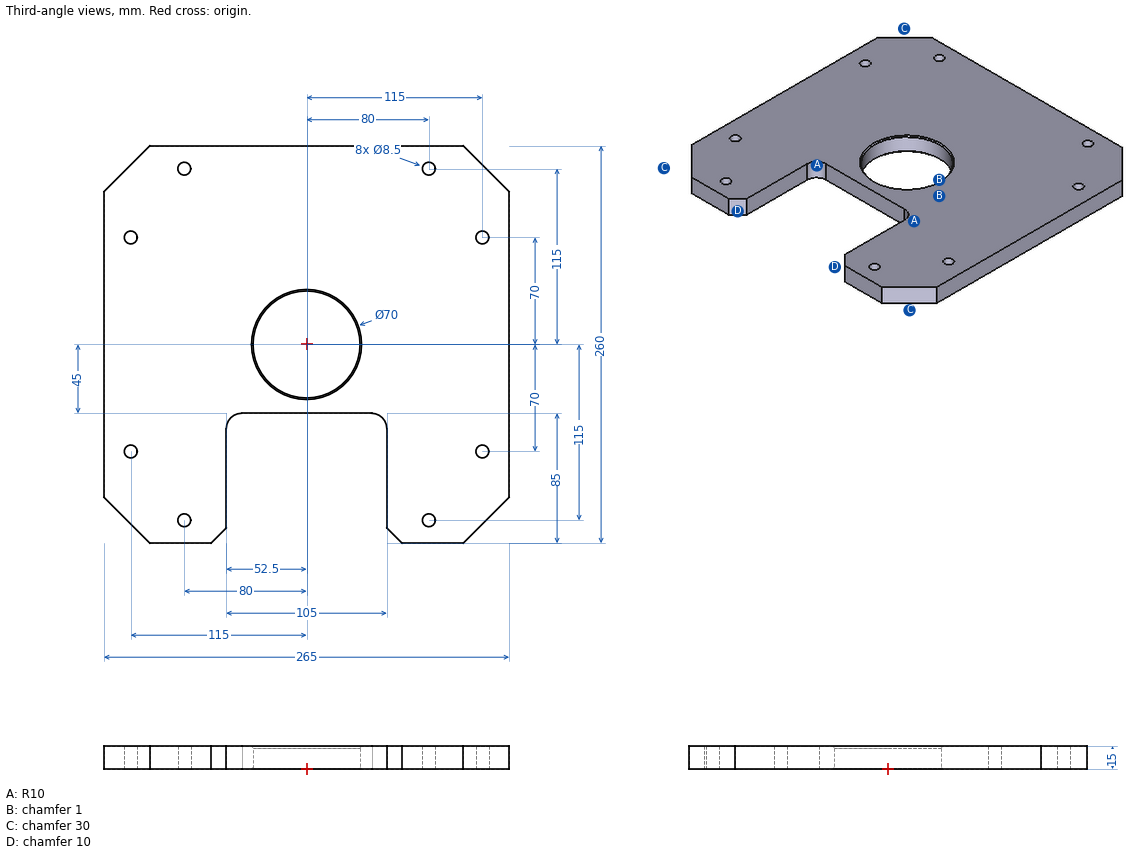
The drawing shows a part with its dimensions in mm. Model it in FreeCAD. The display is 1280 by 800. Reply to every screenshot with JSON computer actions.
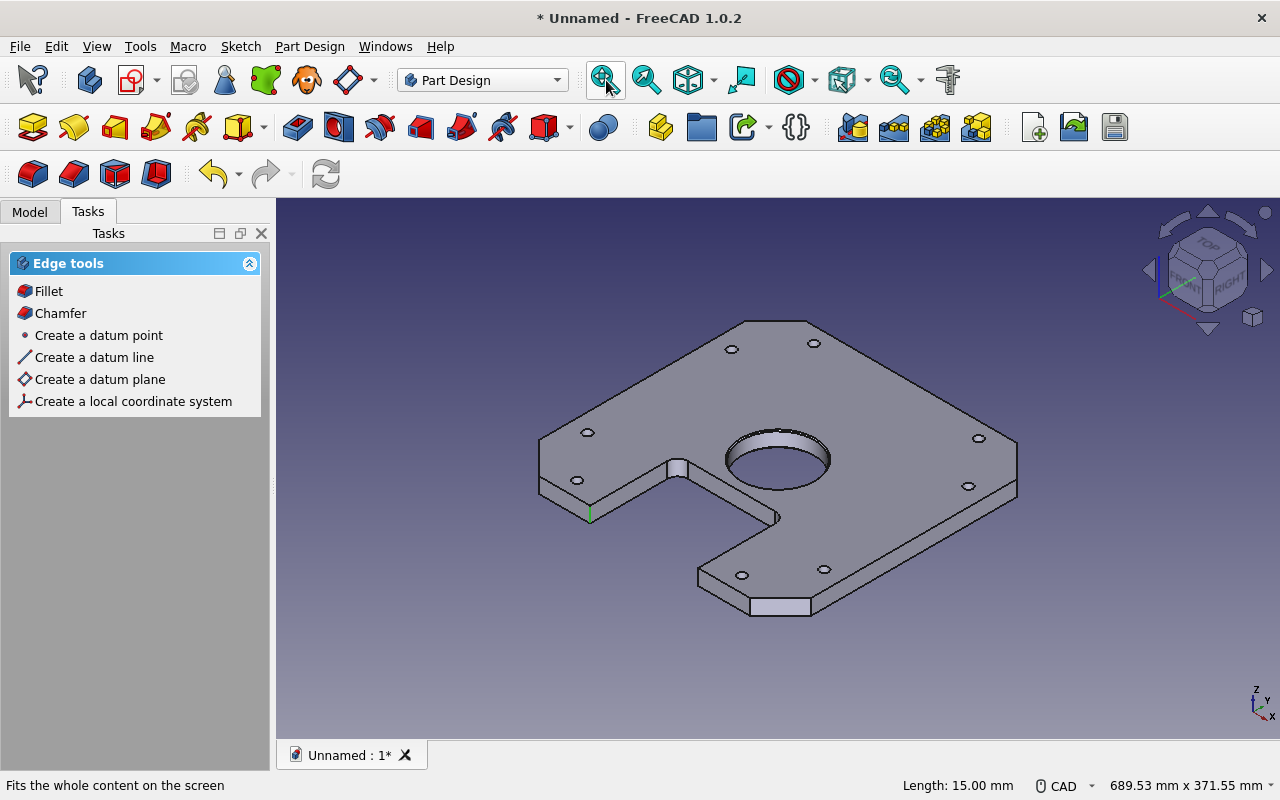
{"action": "key", "text": "2"}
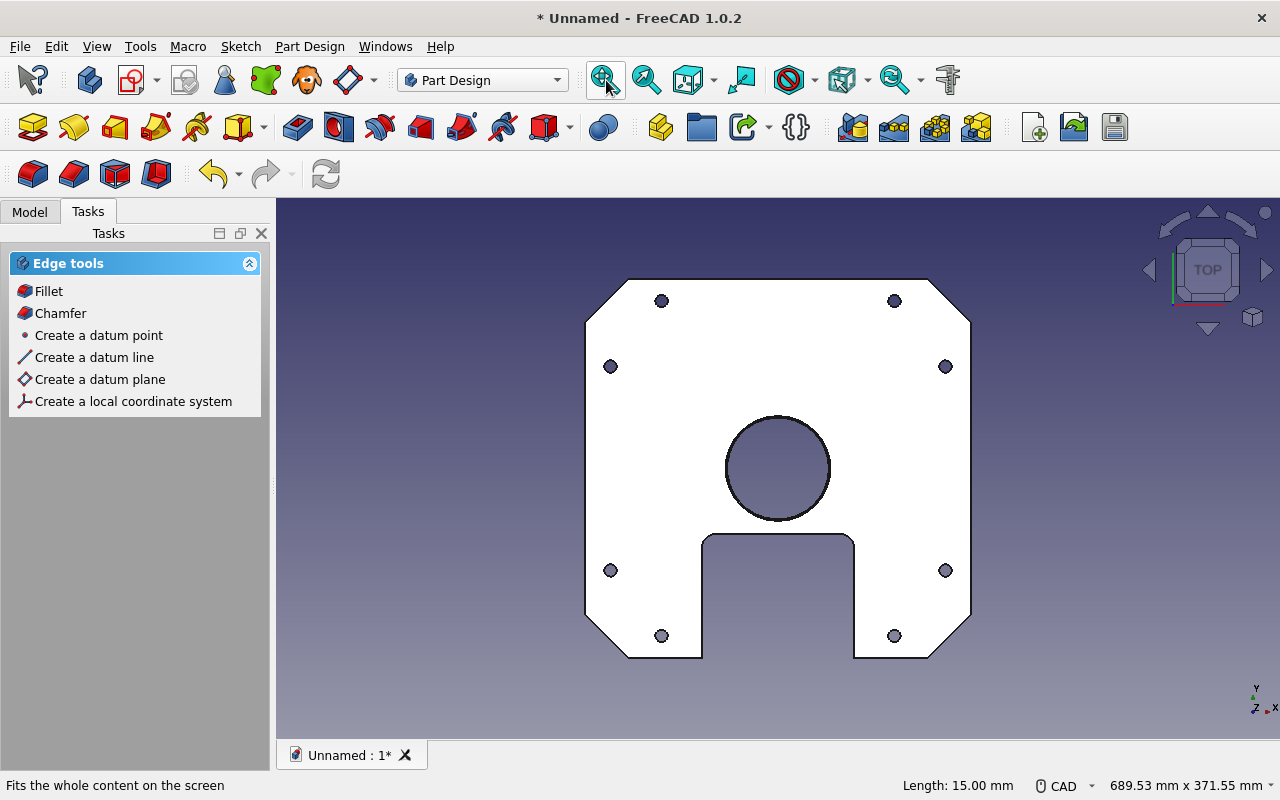
{"action": "scroll", "coordinate": [854, 657], "scroll_direction": "up", "scroll_amount": 4}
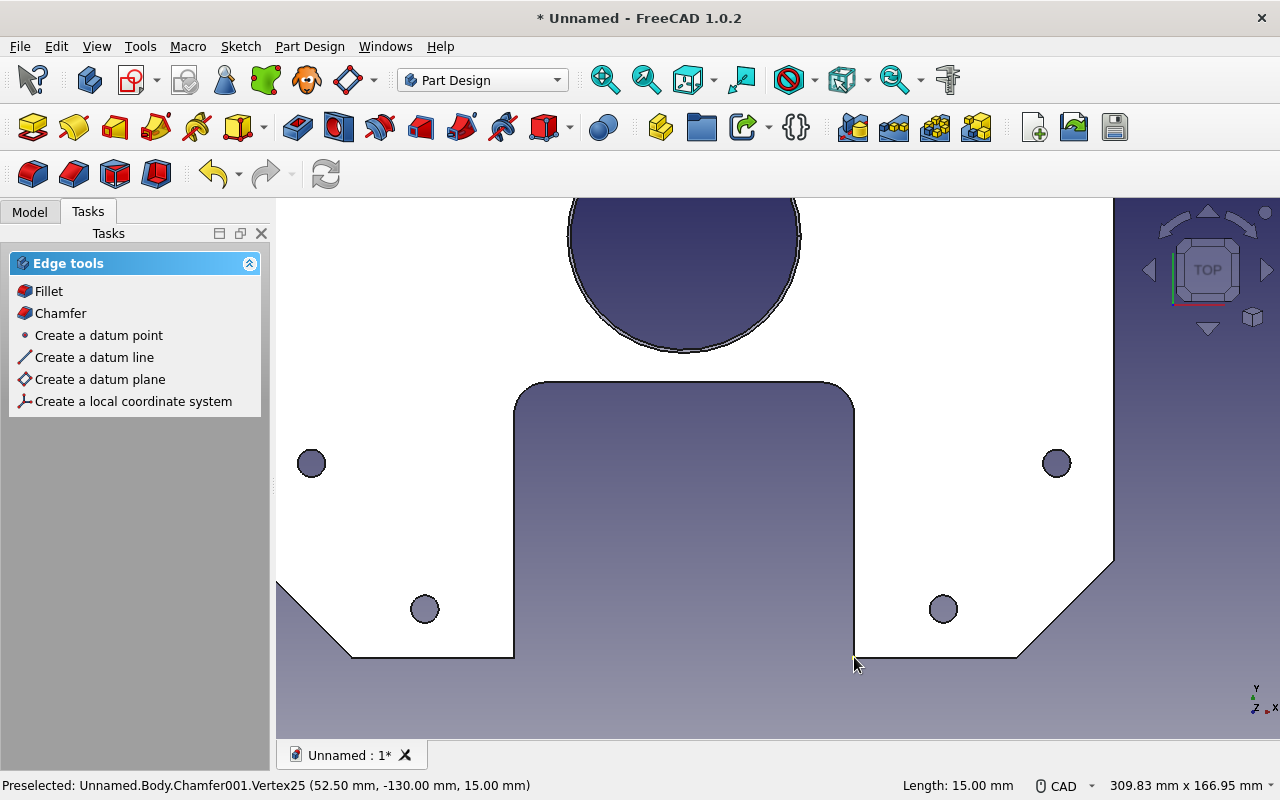
{"action": "left_click", "coordinate": [606, 80]}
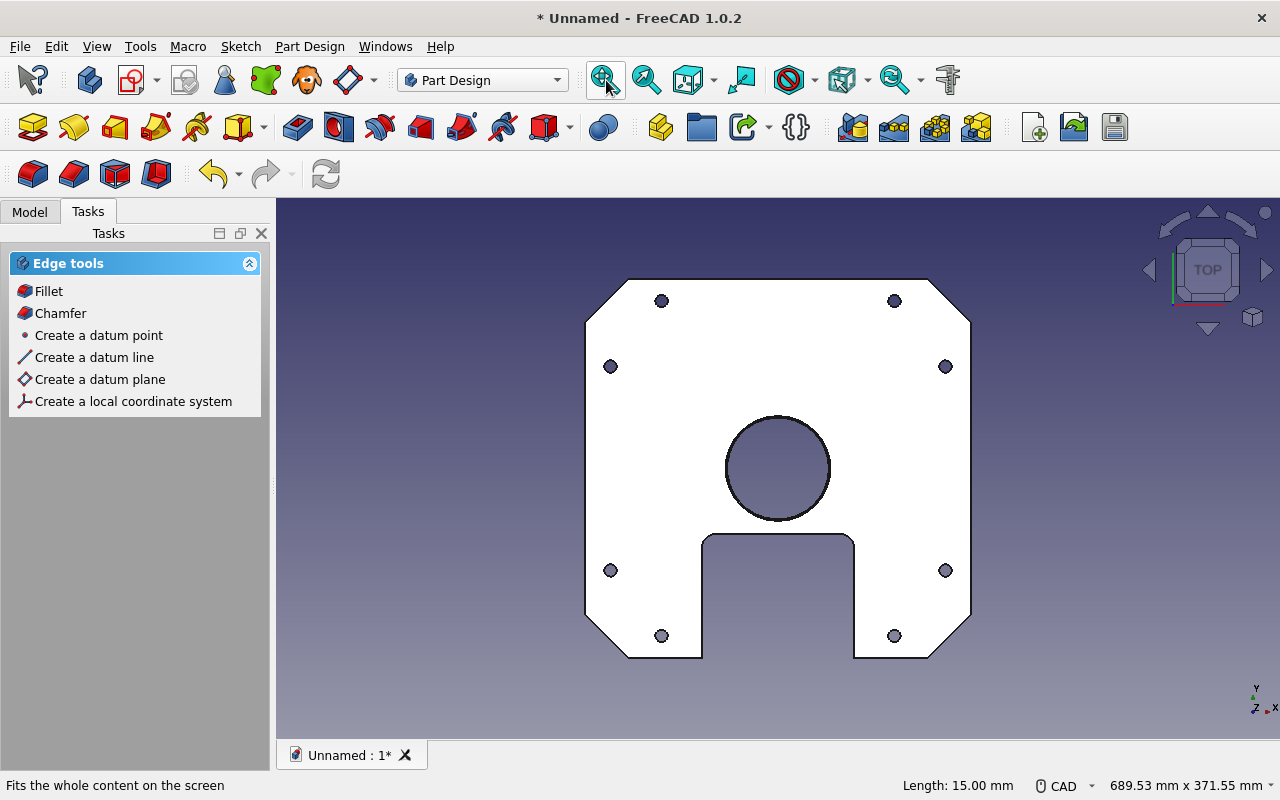
{"action": "key", "text": "1"}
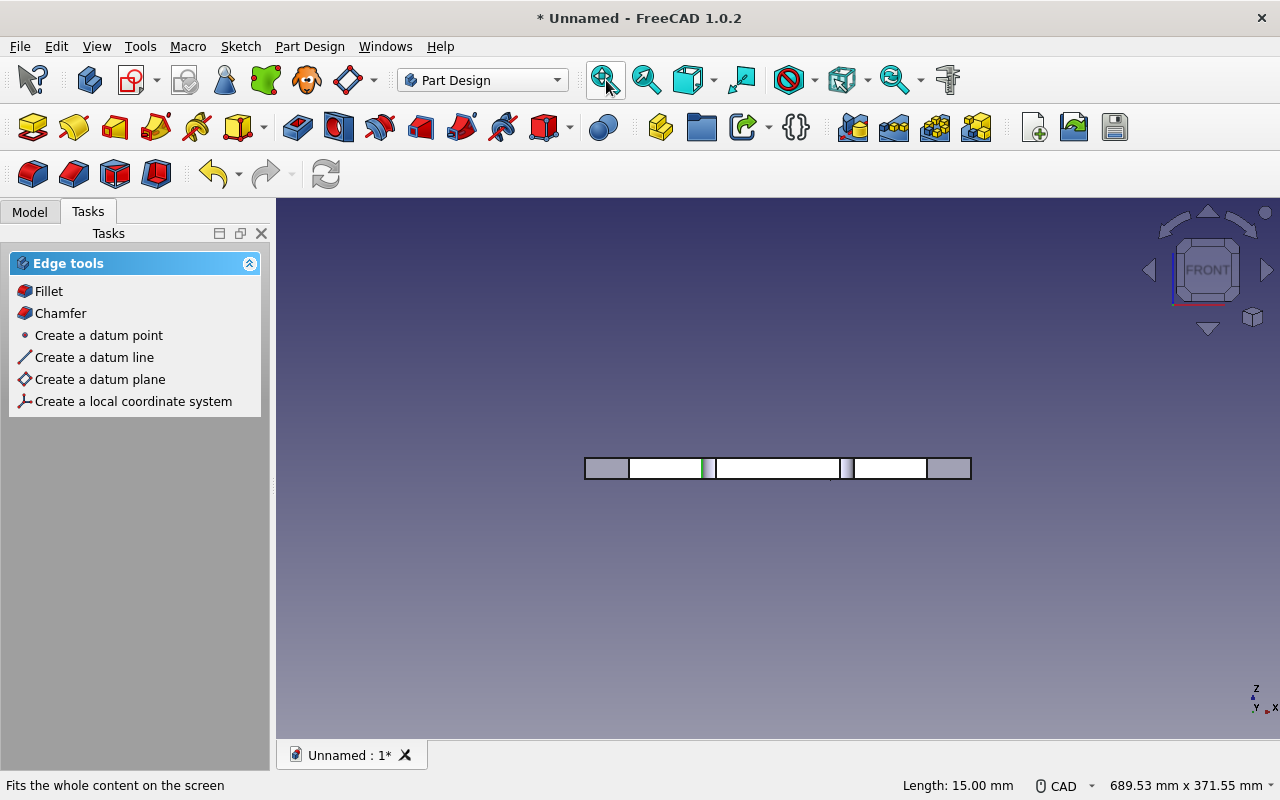
{"action": "key", "text": "v f"}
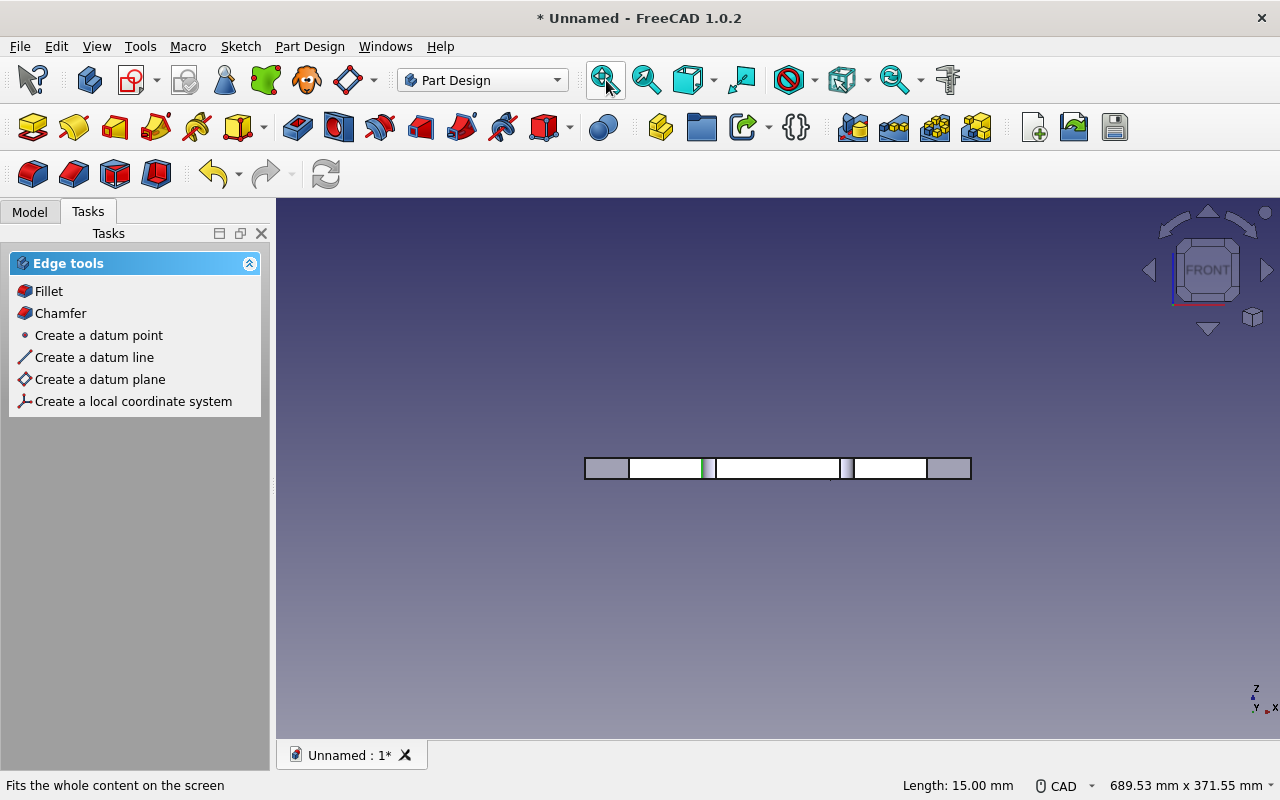
{"action": "left_click", "coordinate": [854, 468], "text": "ctrl"}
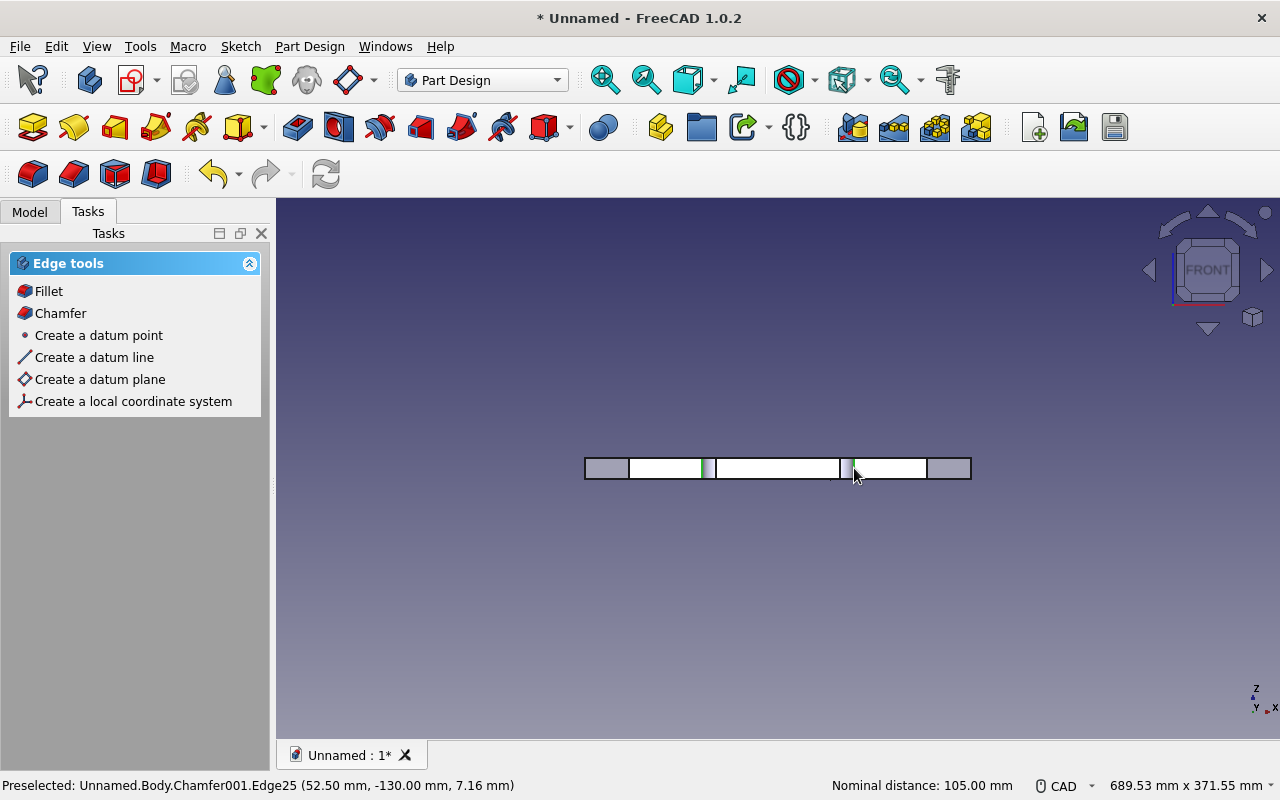
{"action": "left_click", "coordinate": [74, 174]}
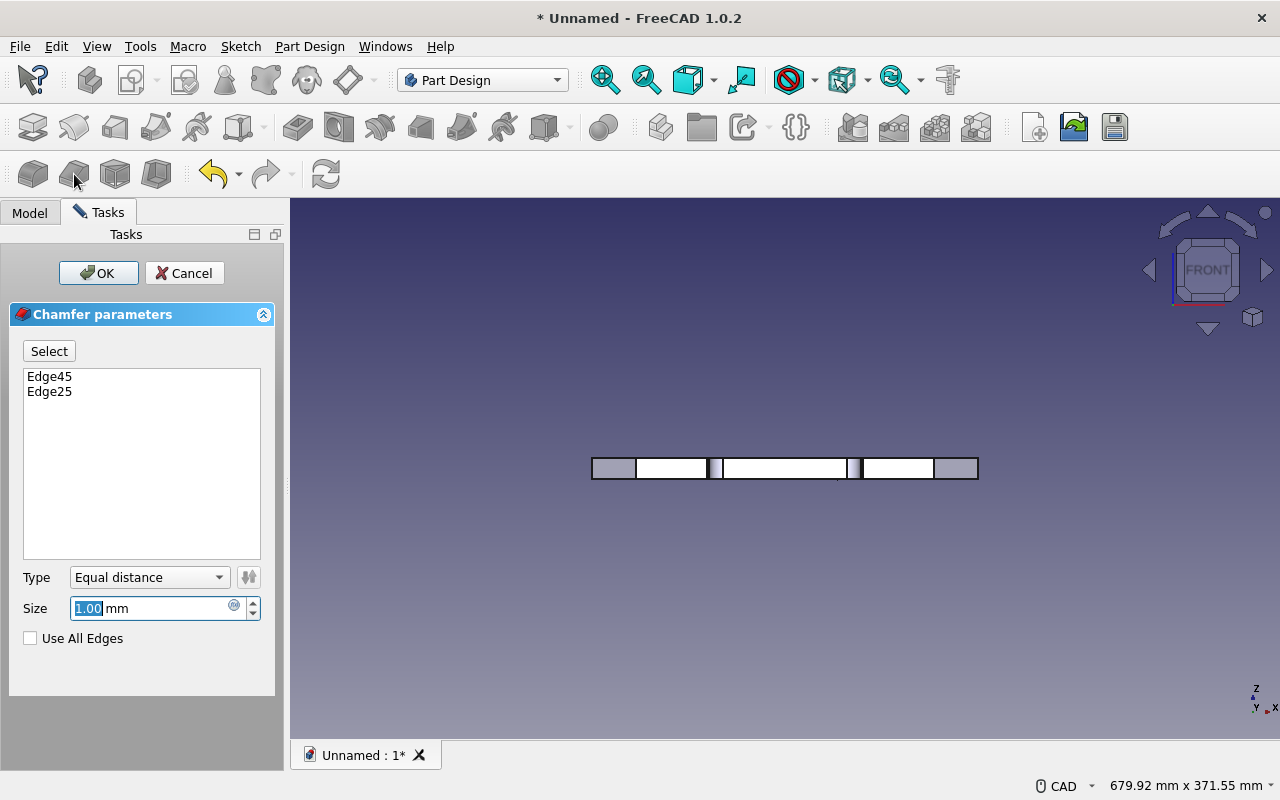
{"action": "type", "text": "10"}
{"action": "key", "text": "Tab"}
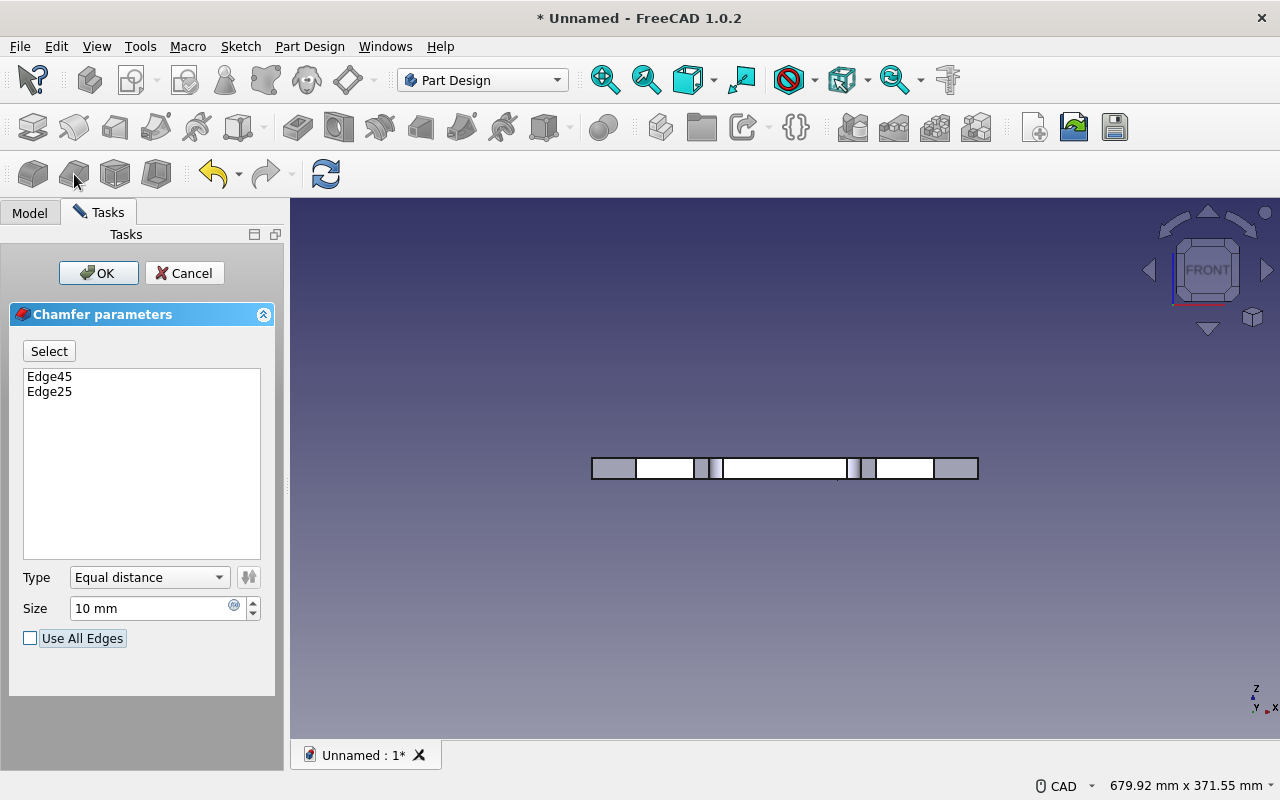
{"action": "left_click", "coordinate": [99, 273]}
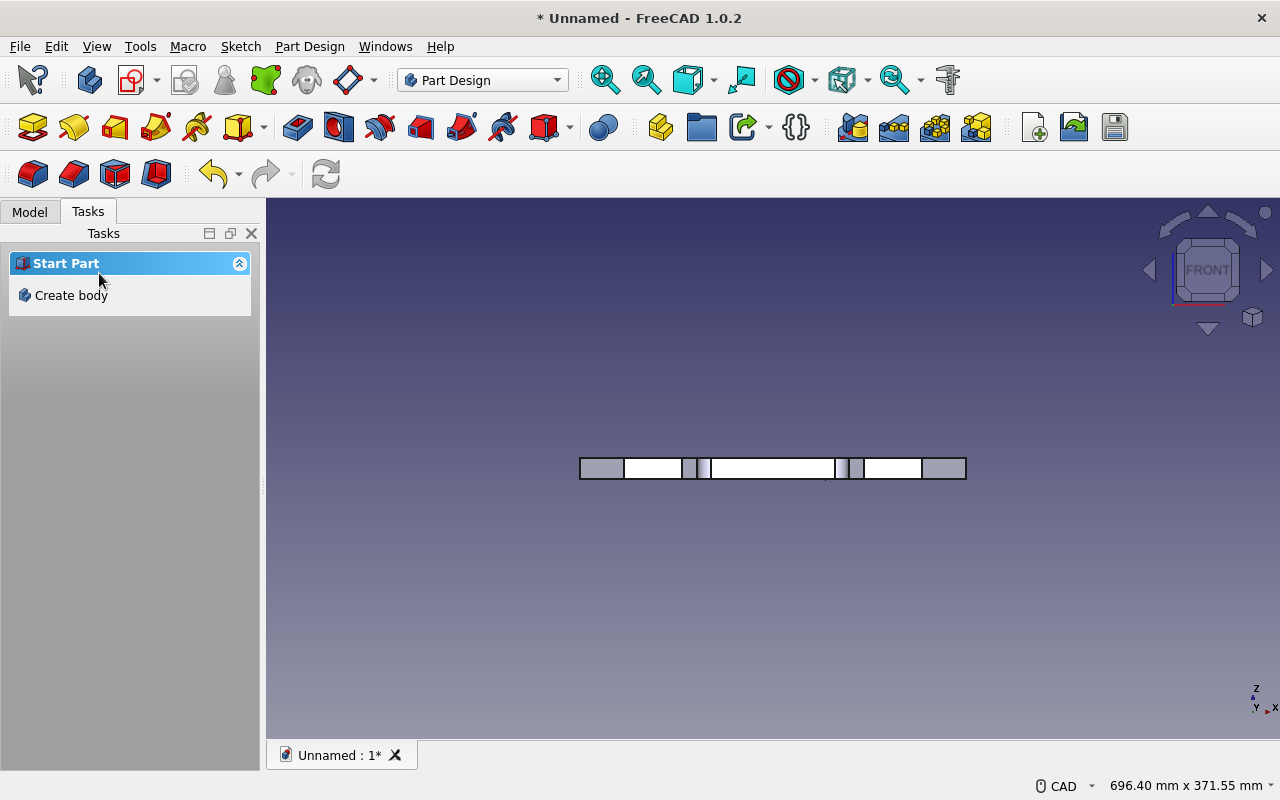
{"action": "key", "text": "0"}